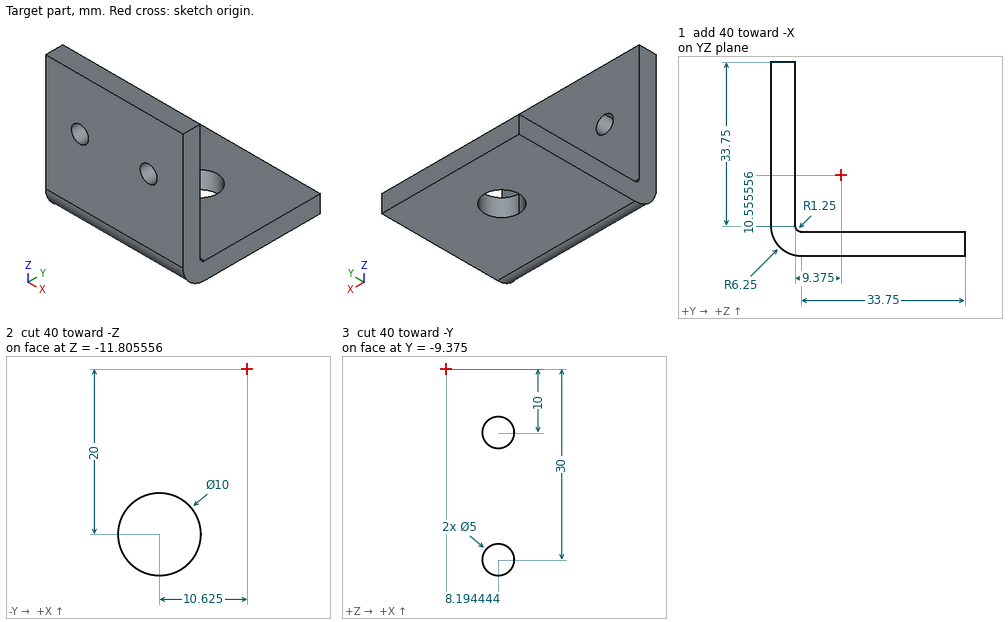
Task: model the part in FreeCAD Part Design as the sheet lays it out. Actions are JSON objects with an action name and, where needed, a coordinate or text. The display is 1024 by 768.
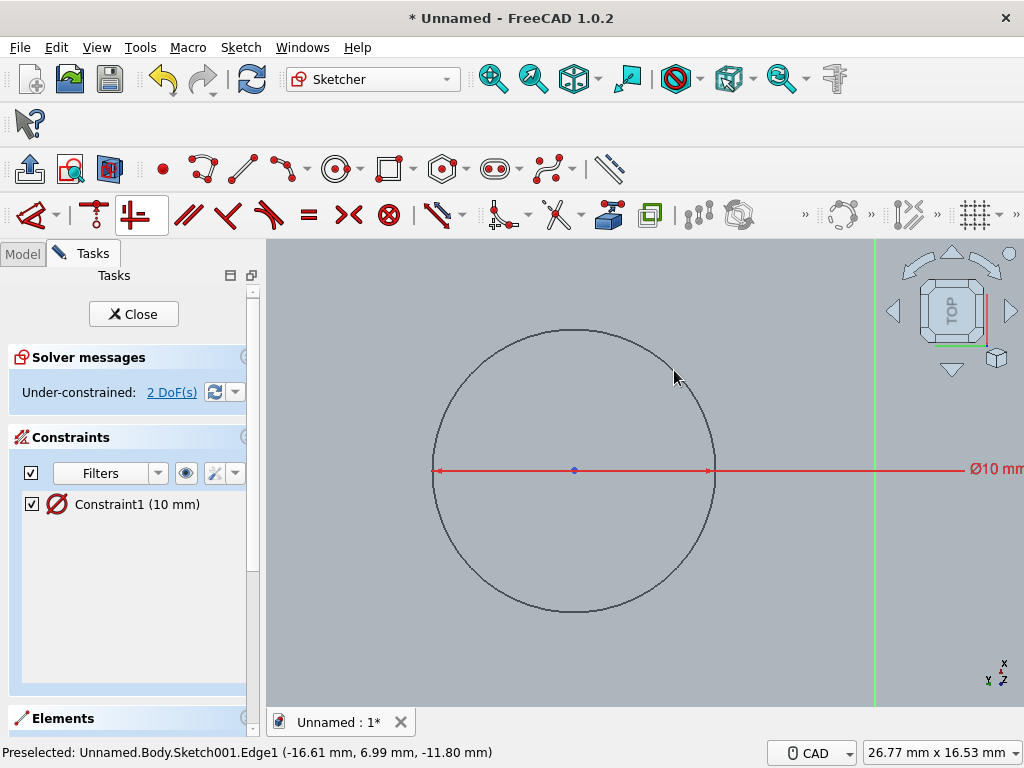
{"action": "key", "text": "d"}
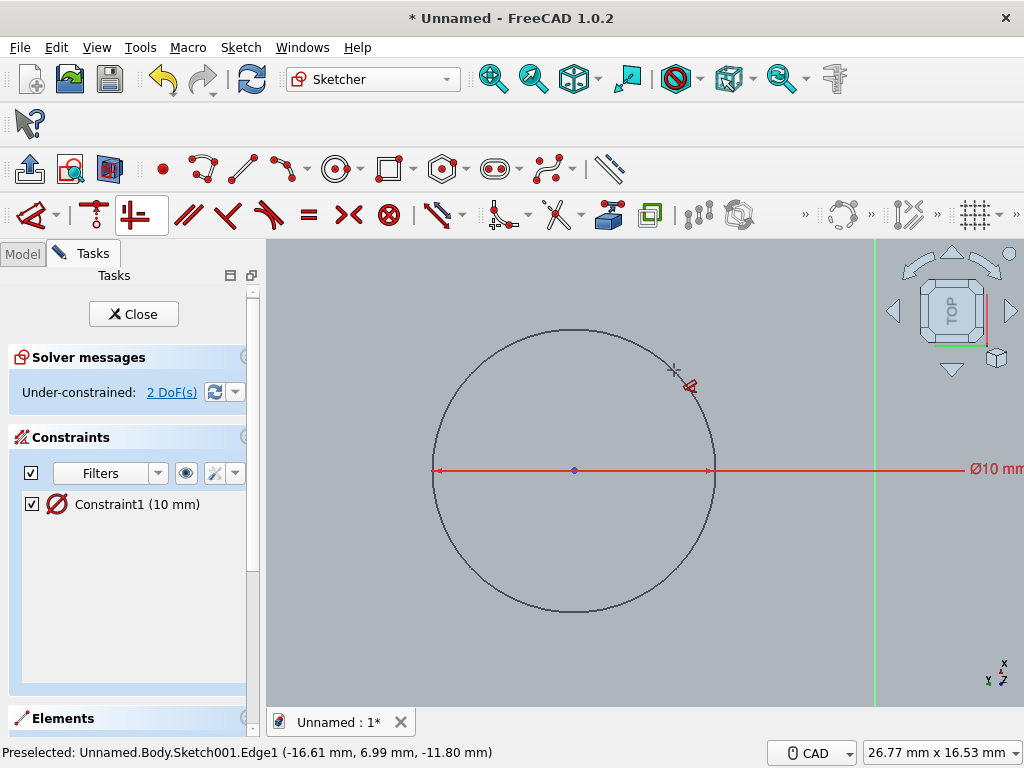
{"action": "left_click", "coordinate": [574, 471]}
{"action": "left_click", "coordinate": [540, 369]}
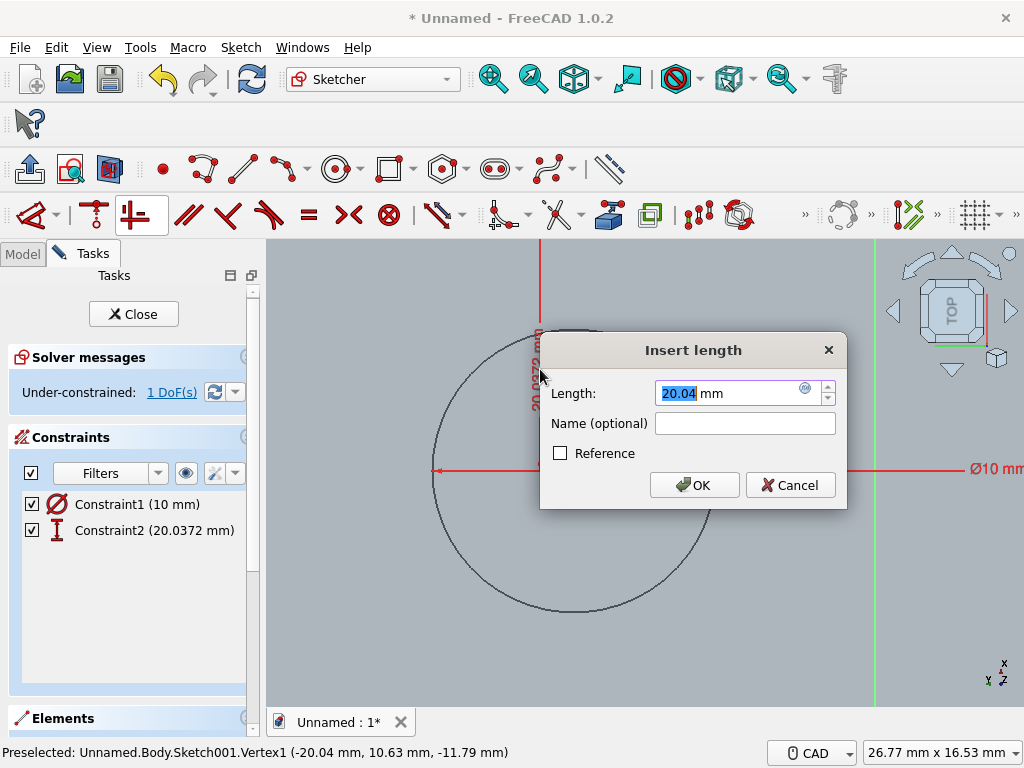
{"action": "type", "text": "20"}
{"action": "key", "text": "Return"}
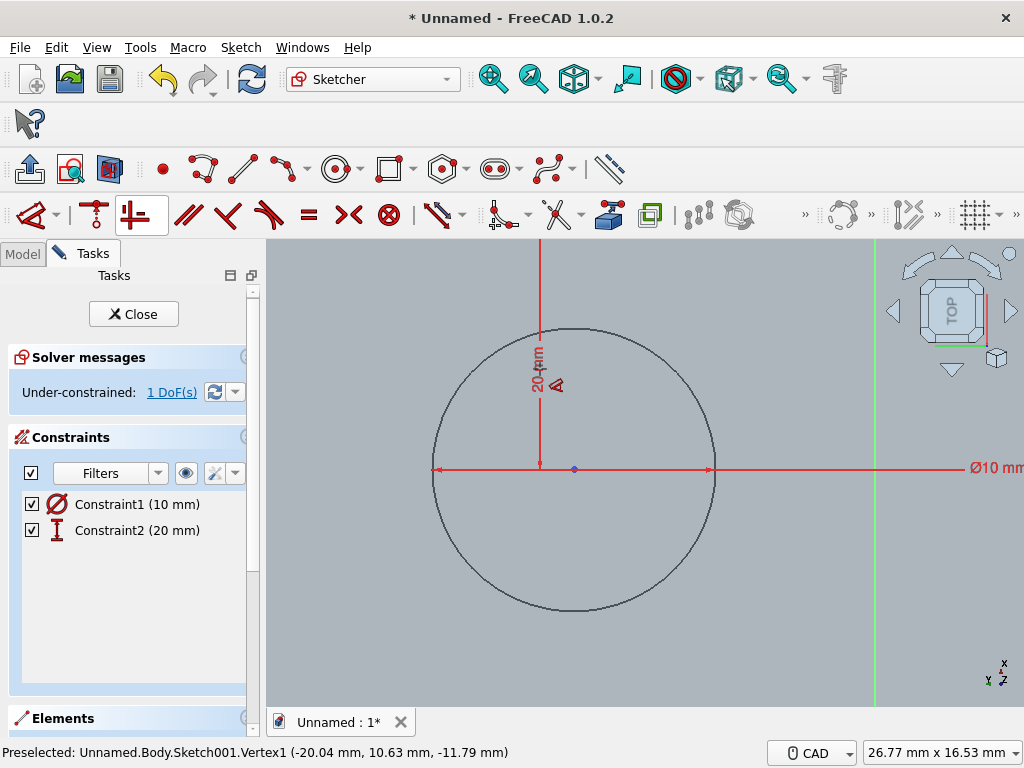
{"action": "left_click", "coordinate": [574, 470]}
{"action": "left_click", "coordinate": [651, 504]}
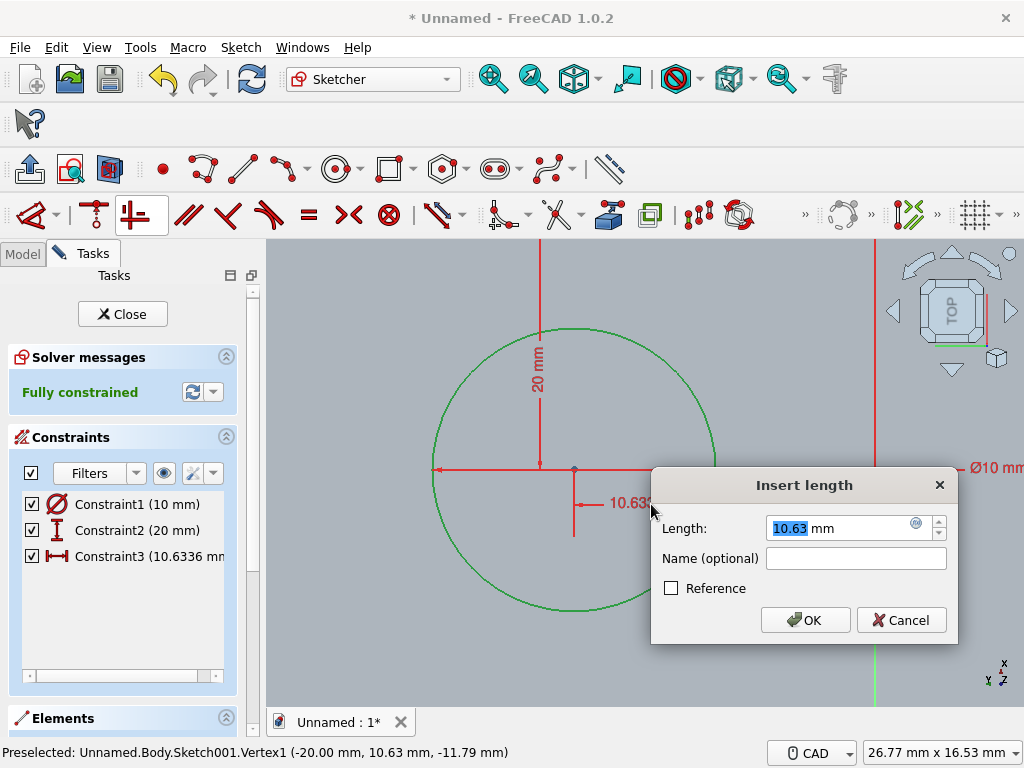
{"action": "type", "text": "10.625"}
{"action": "key", "text": "Return"}
{"action": "key", "text": "Escape"}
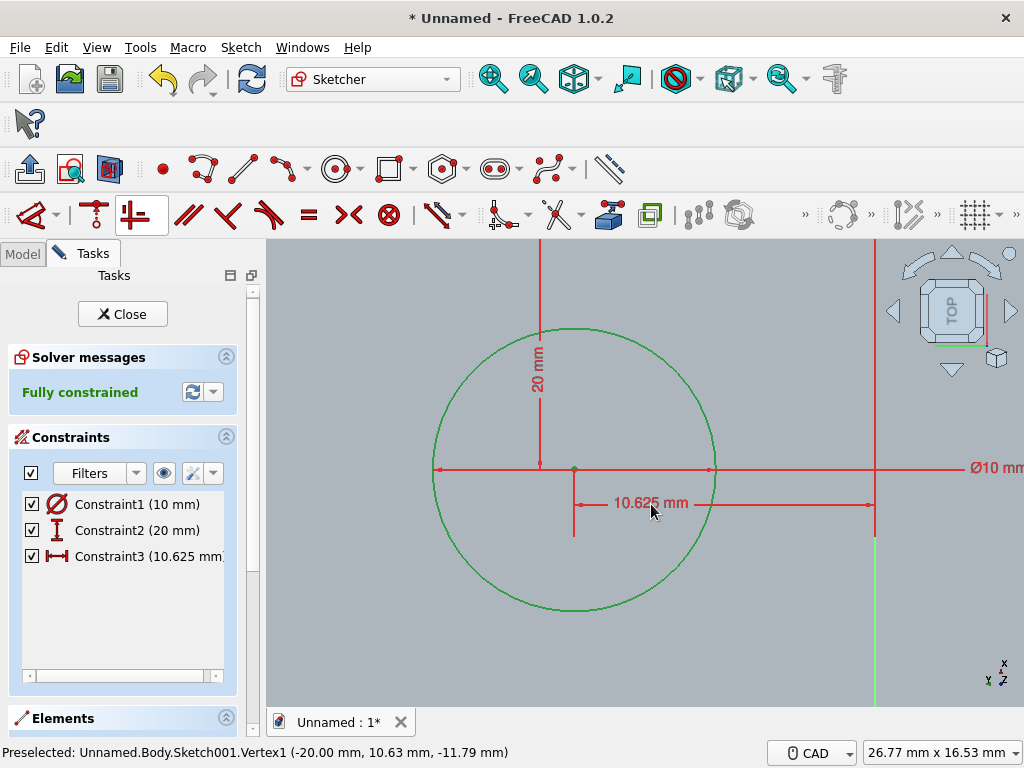
{"action": "left_click", "coordinate": [123, 314]}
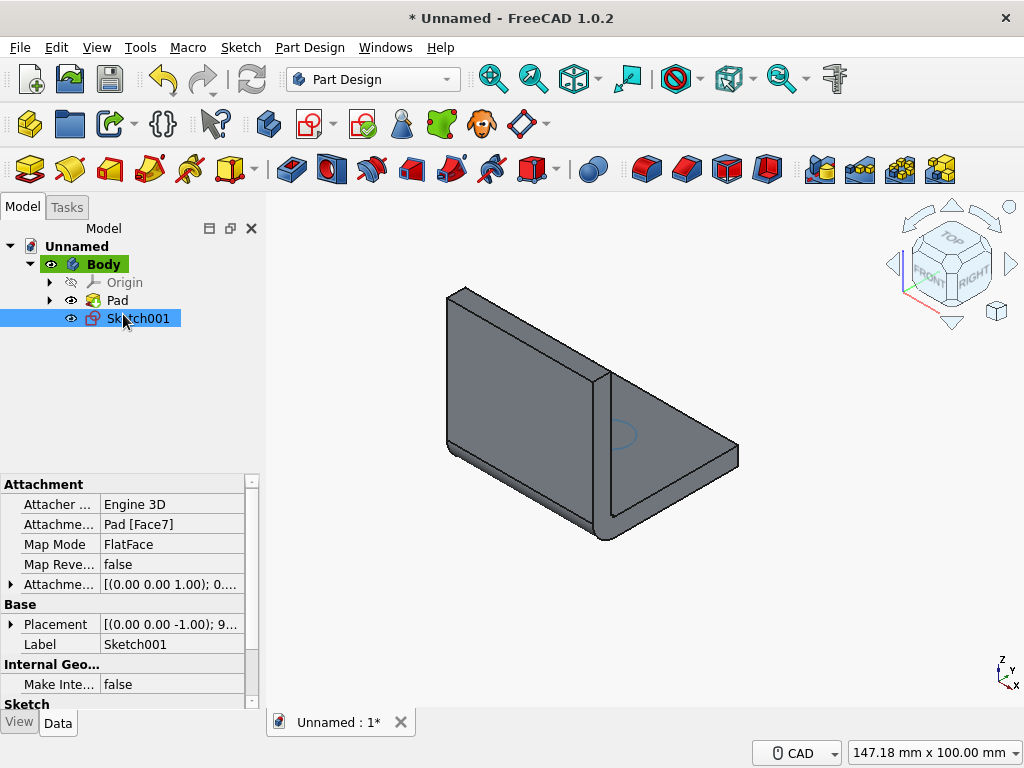
{"action": "left_click", "coordinate": [292, 170]}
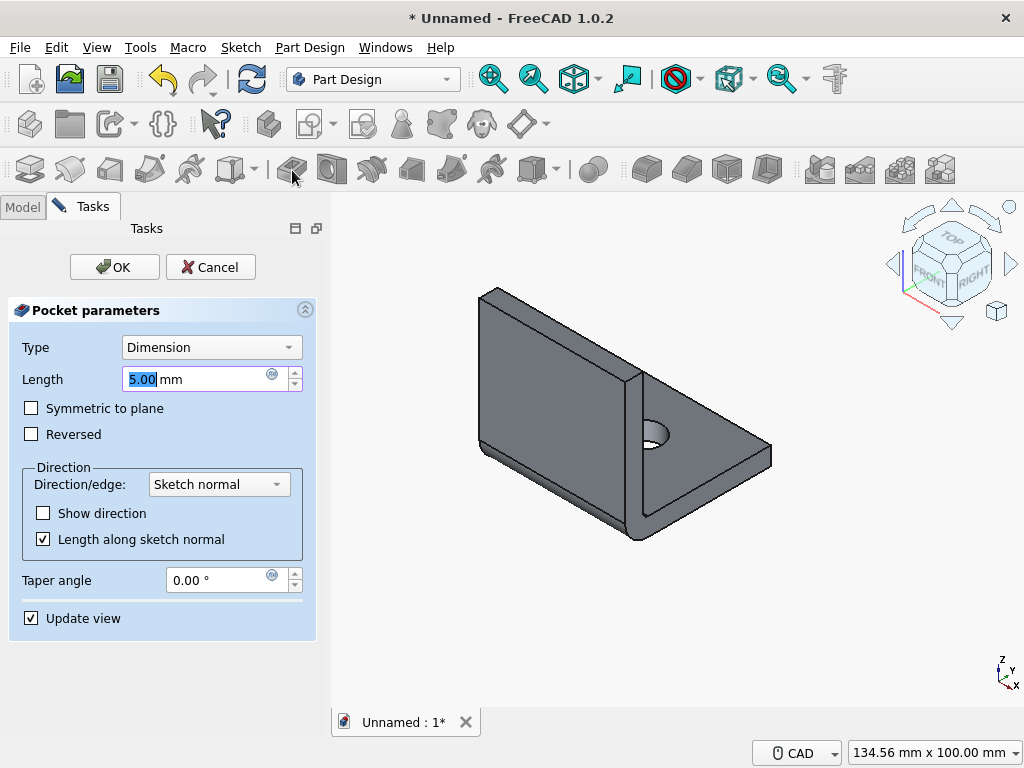
{"action": "type", "text": "40"}
{"action": "key", "text": "Tab"}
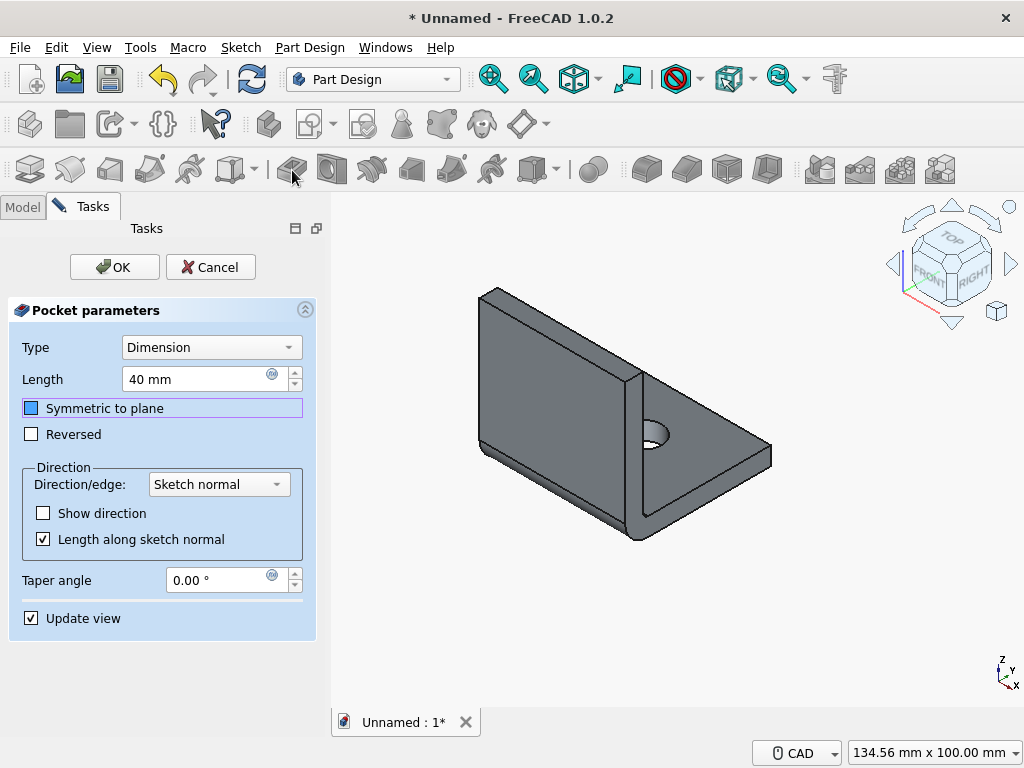
{"action": "left_click", "coordinate": [115, 267]}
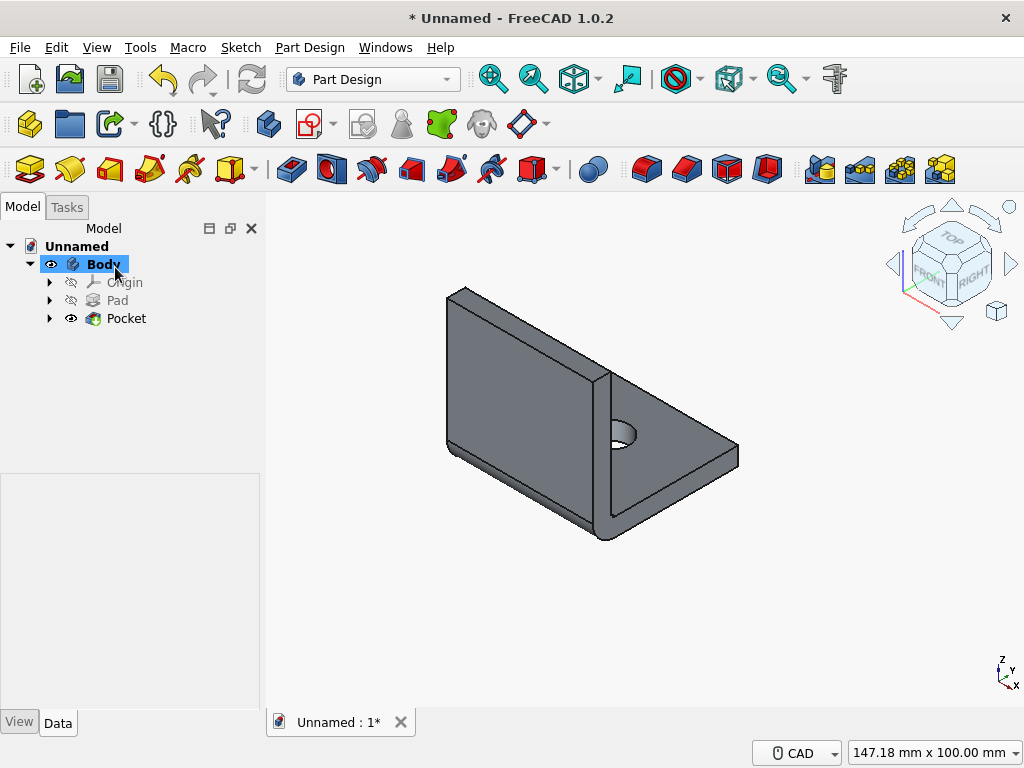
{"action": "key", "text": "4"}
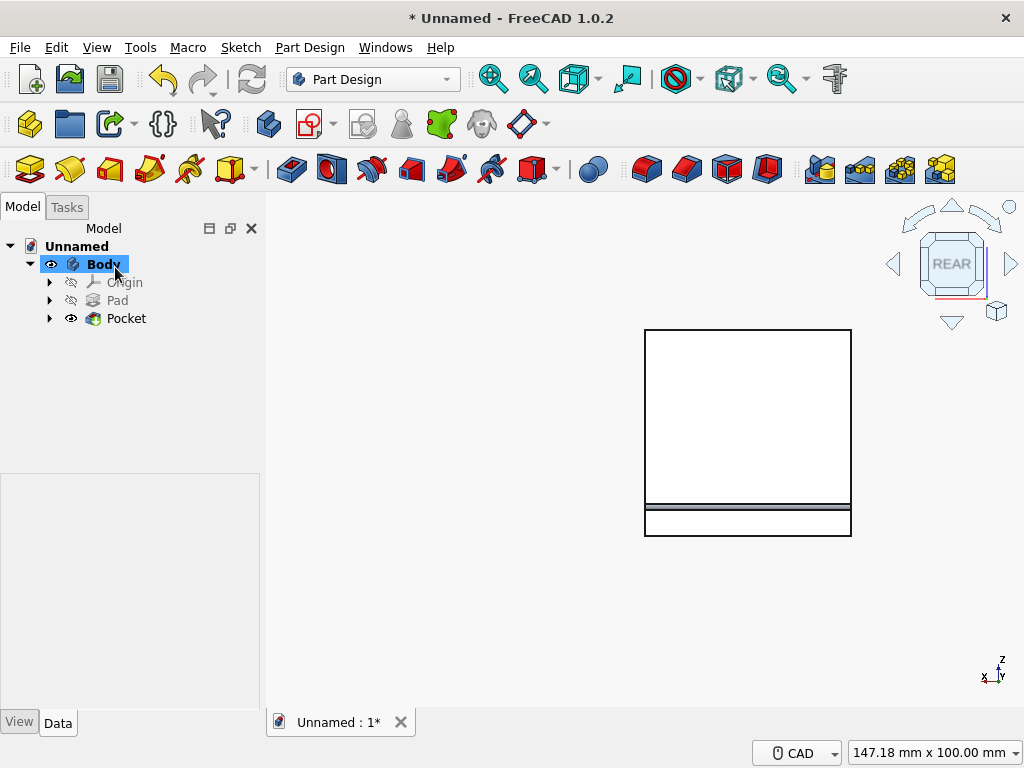
{"action": "key", "text": "v f"}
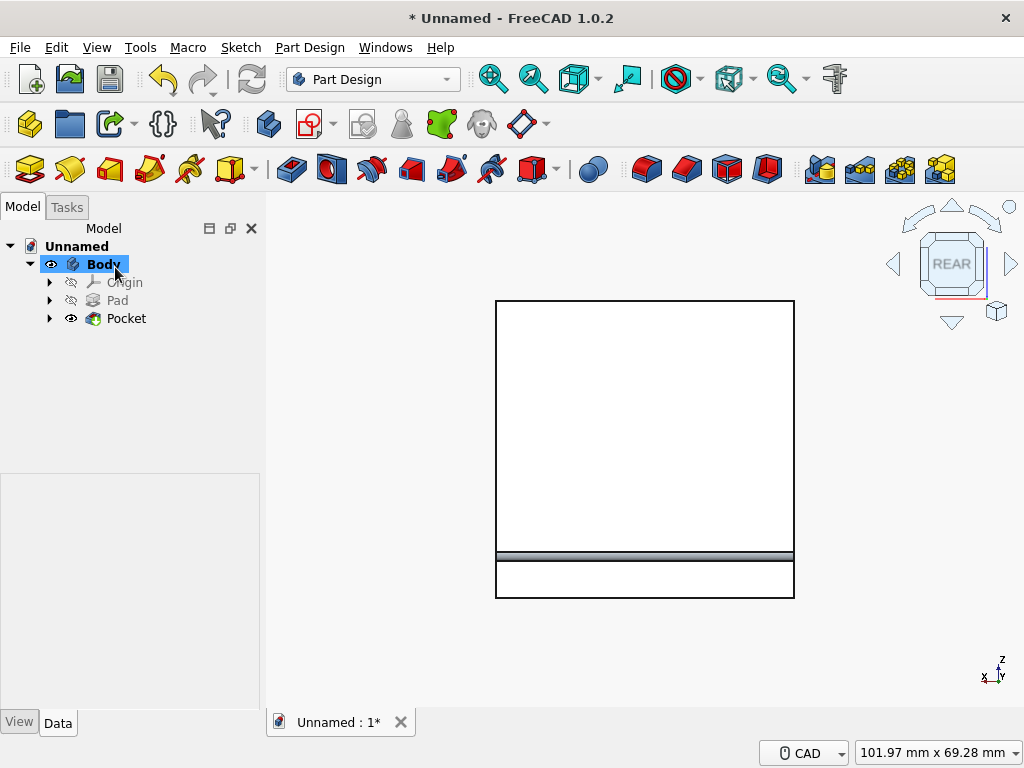
{"action": "left_click", "coordinate": [645, 425]}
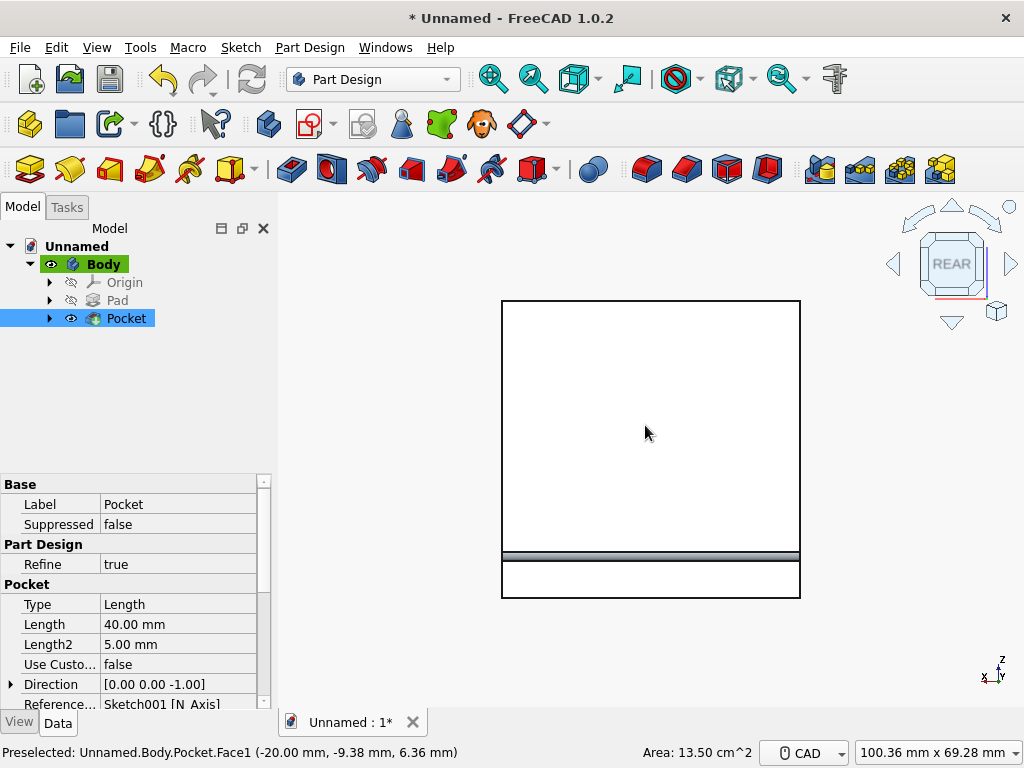
{"action": "left_click", "coordinate": [310, 124]}